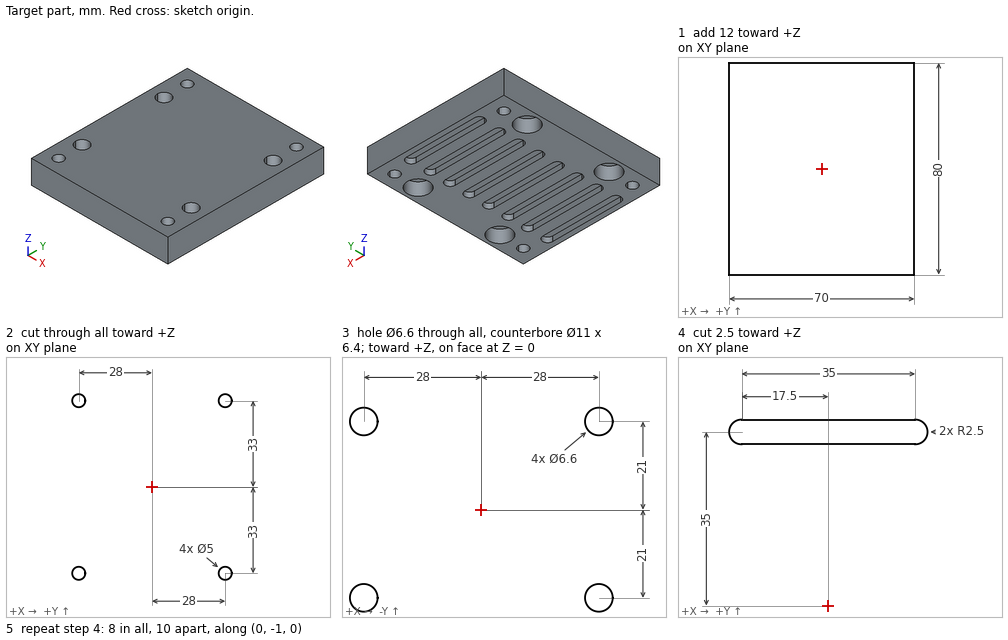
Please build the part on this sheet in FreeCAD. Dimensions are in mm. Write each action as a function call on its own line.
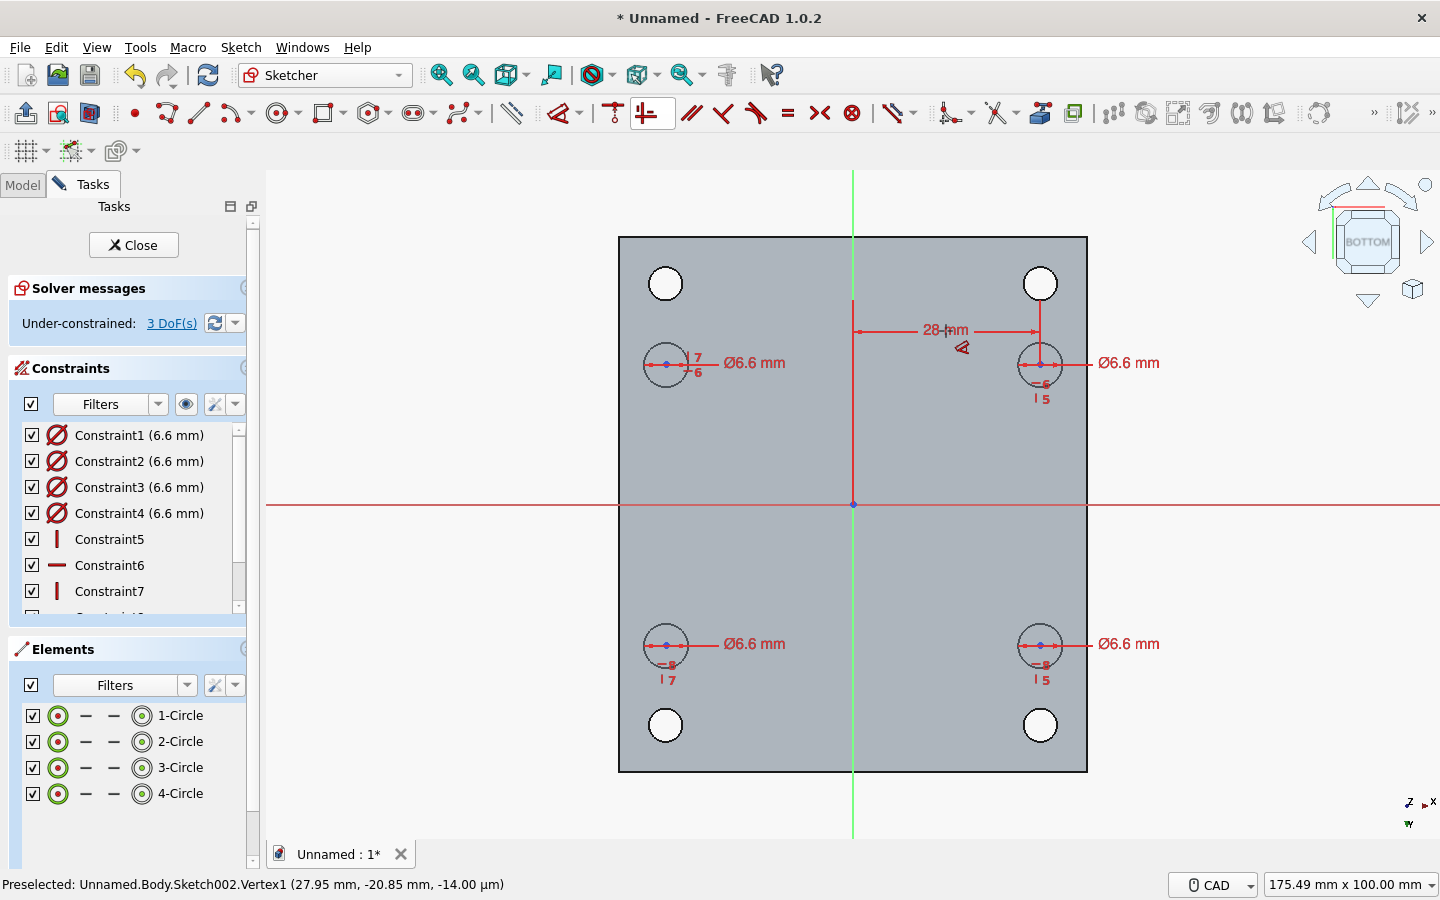
click(1040, 365)
click(1074, 435)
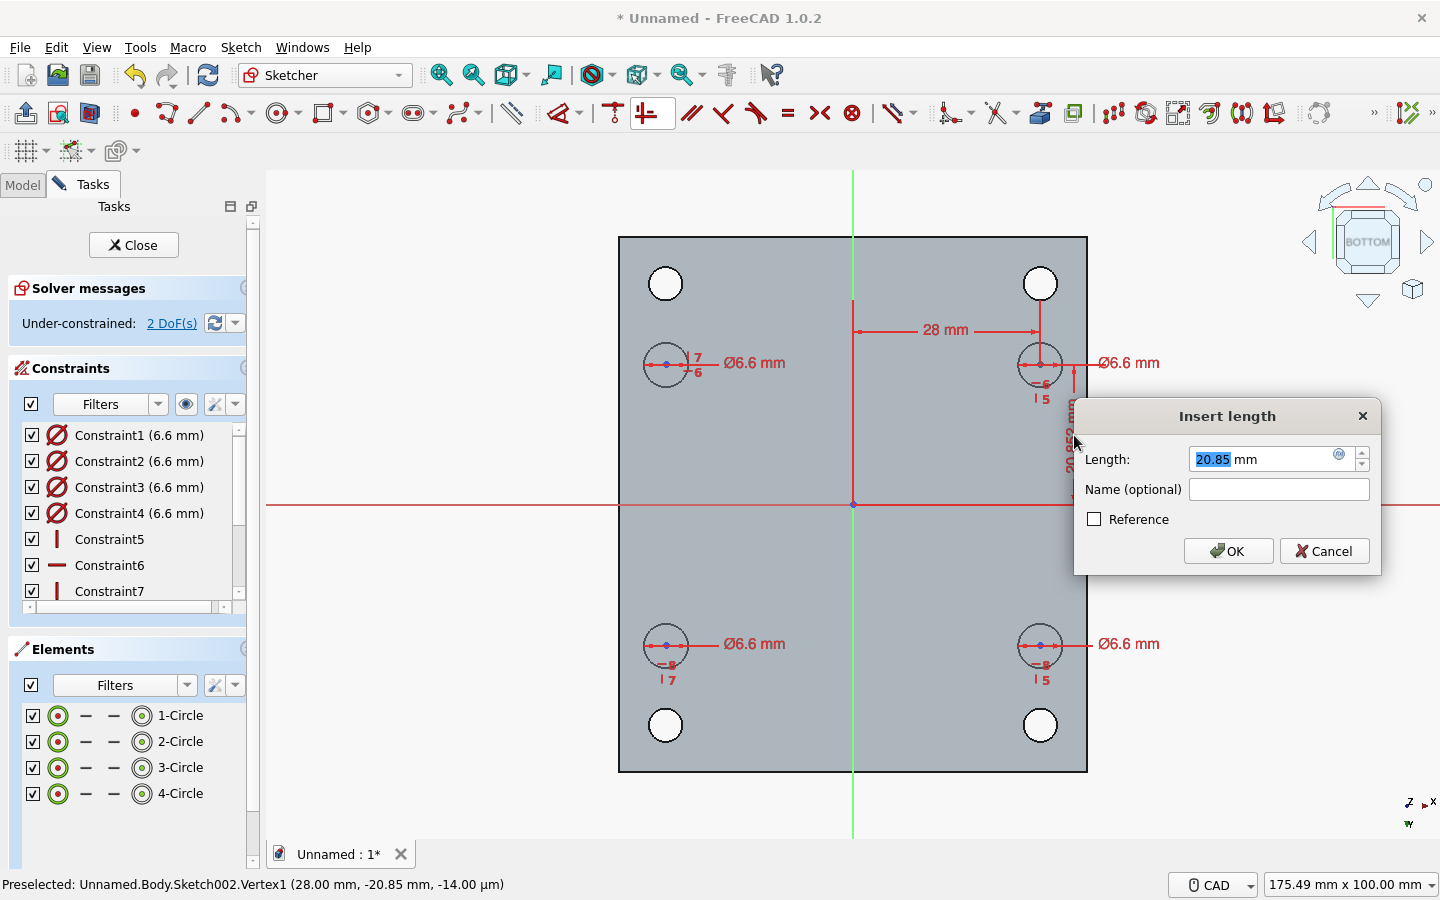
text(21)
key(Return)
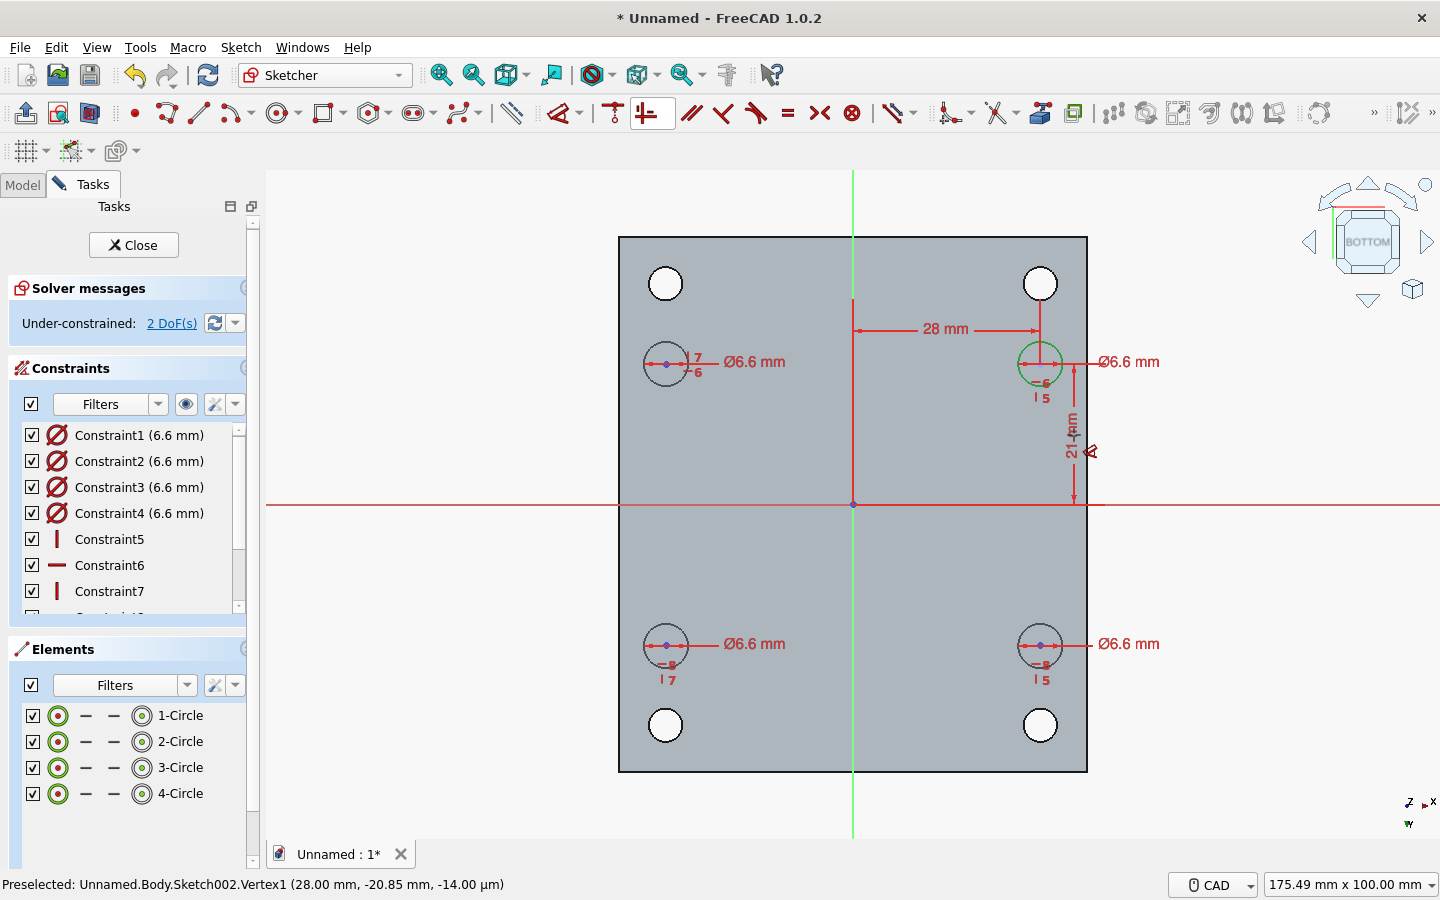
click(1040, 646)
click(1074, 575)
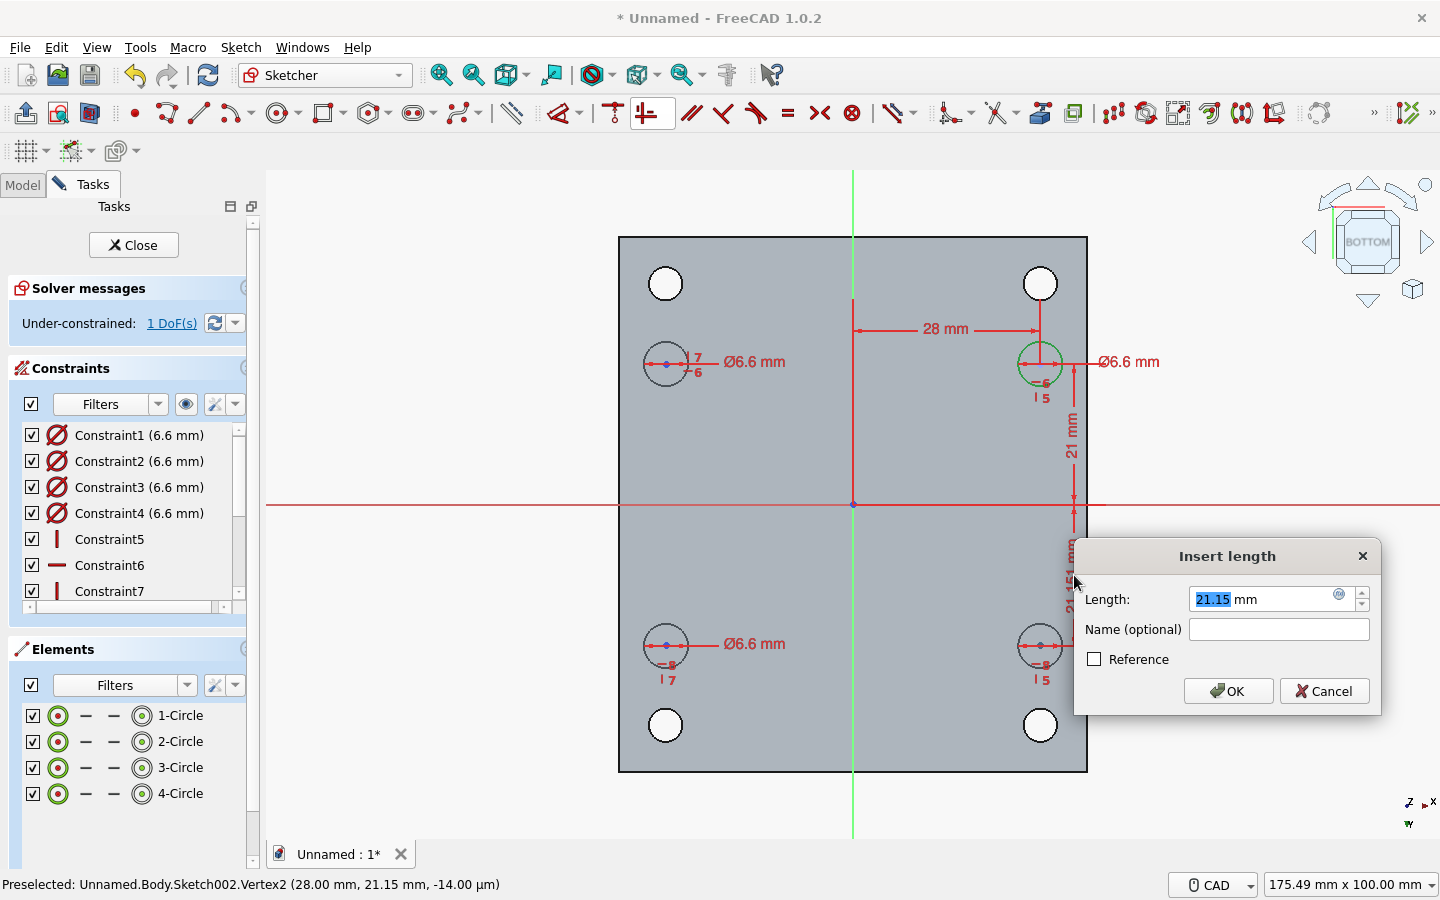
text(21)
key(Return)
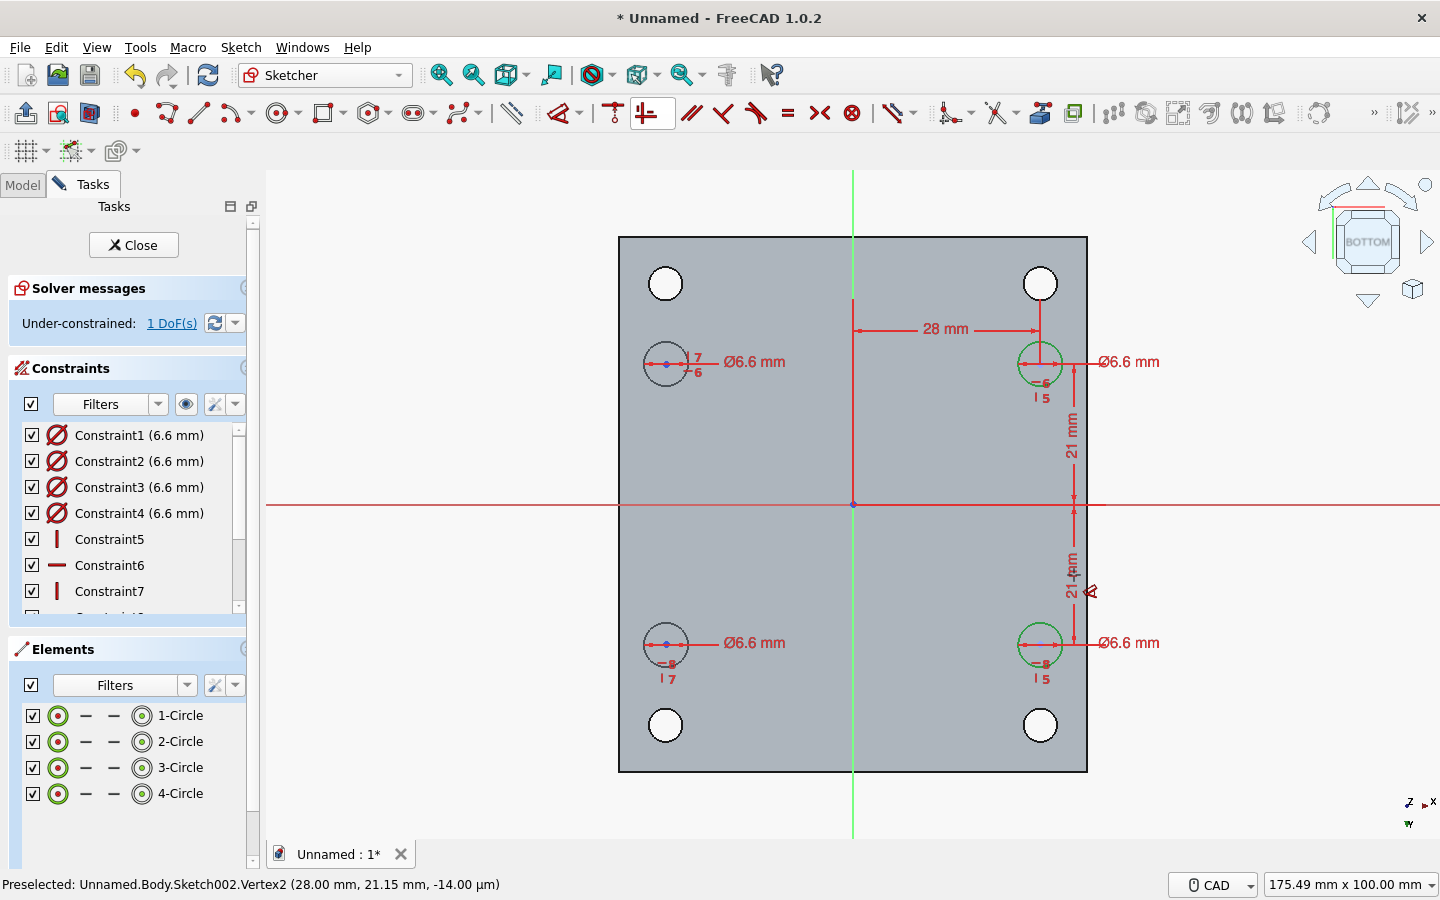
click(666, 364)
click(759, 330)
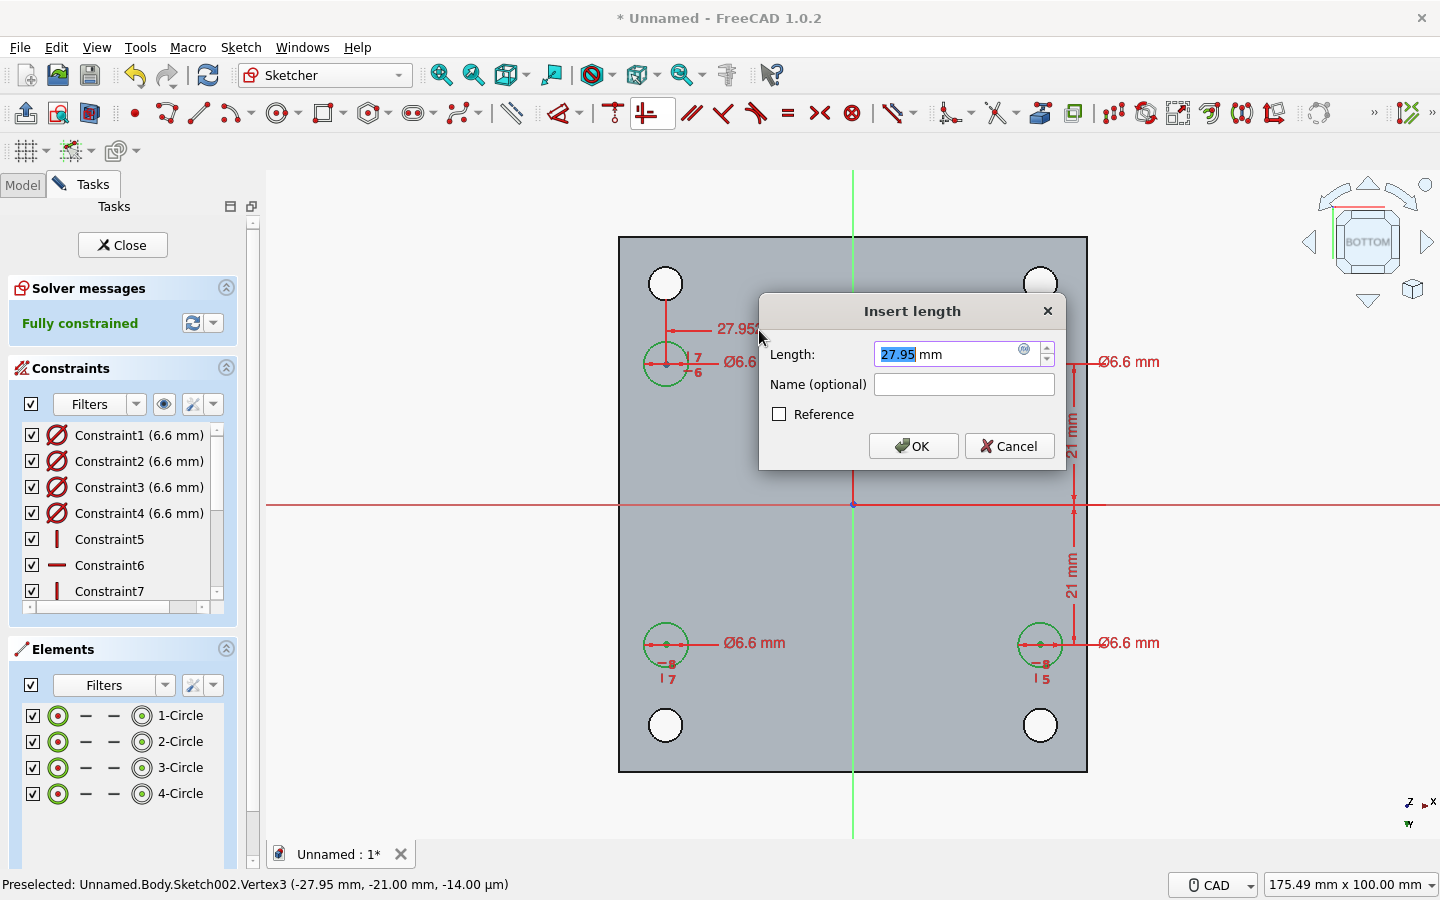
text(28)
key(Return)
key(Escape)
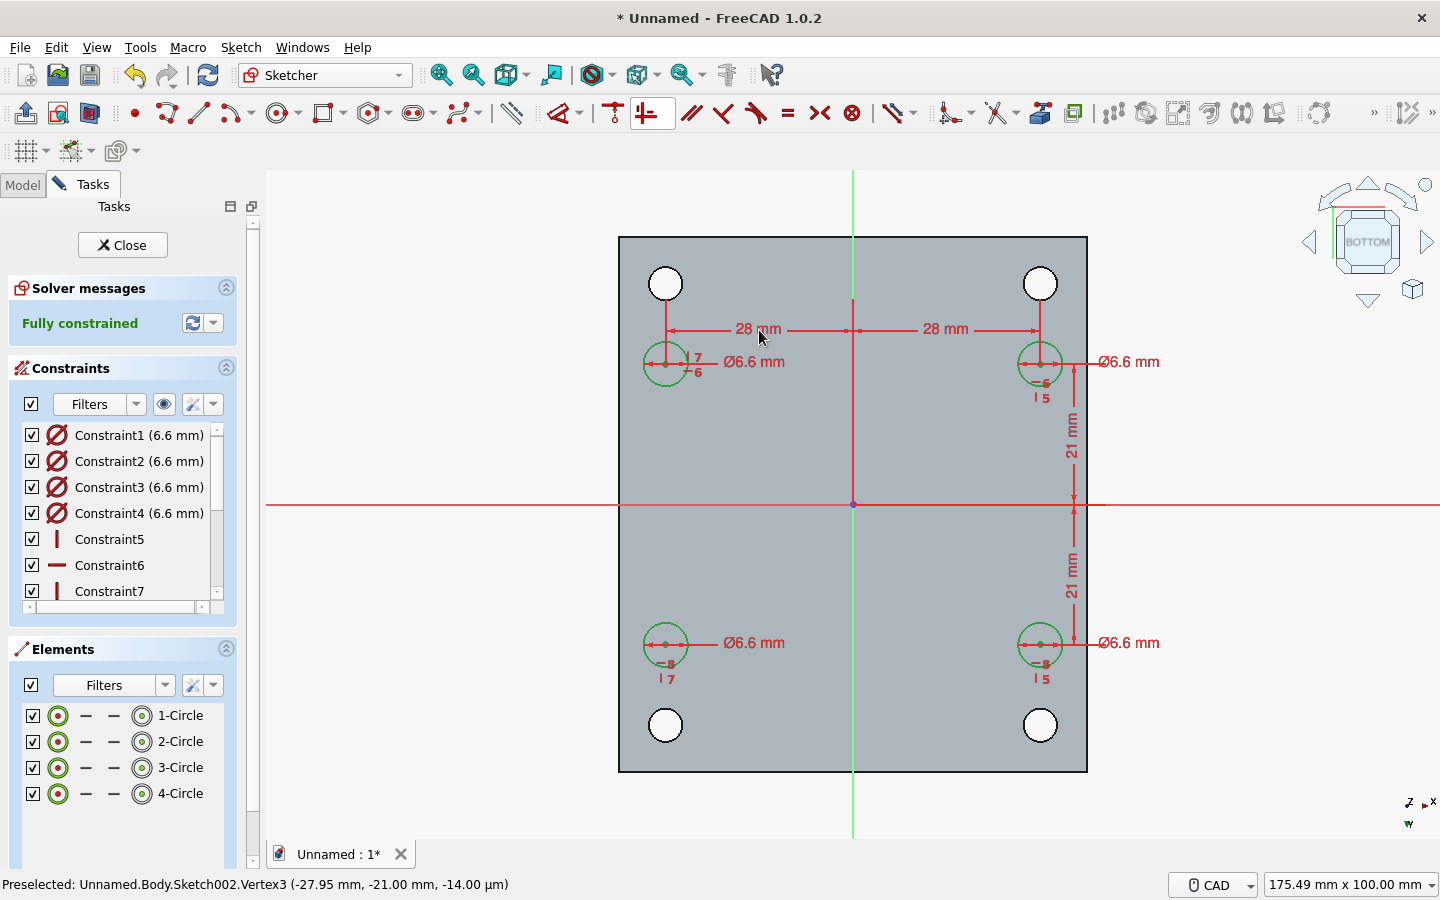
click(123, 245)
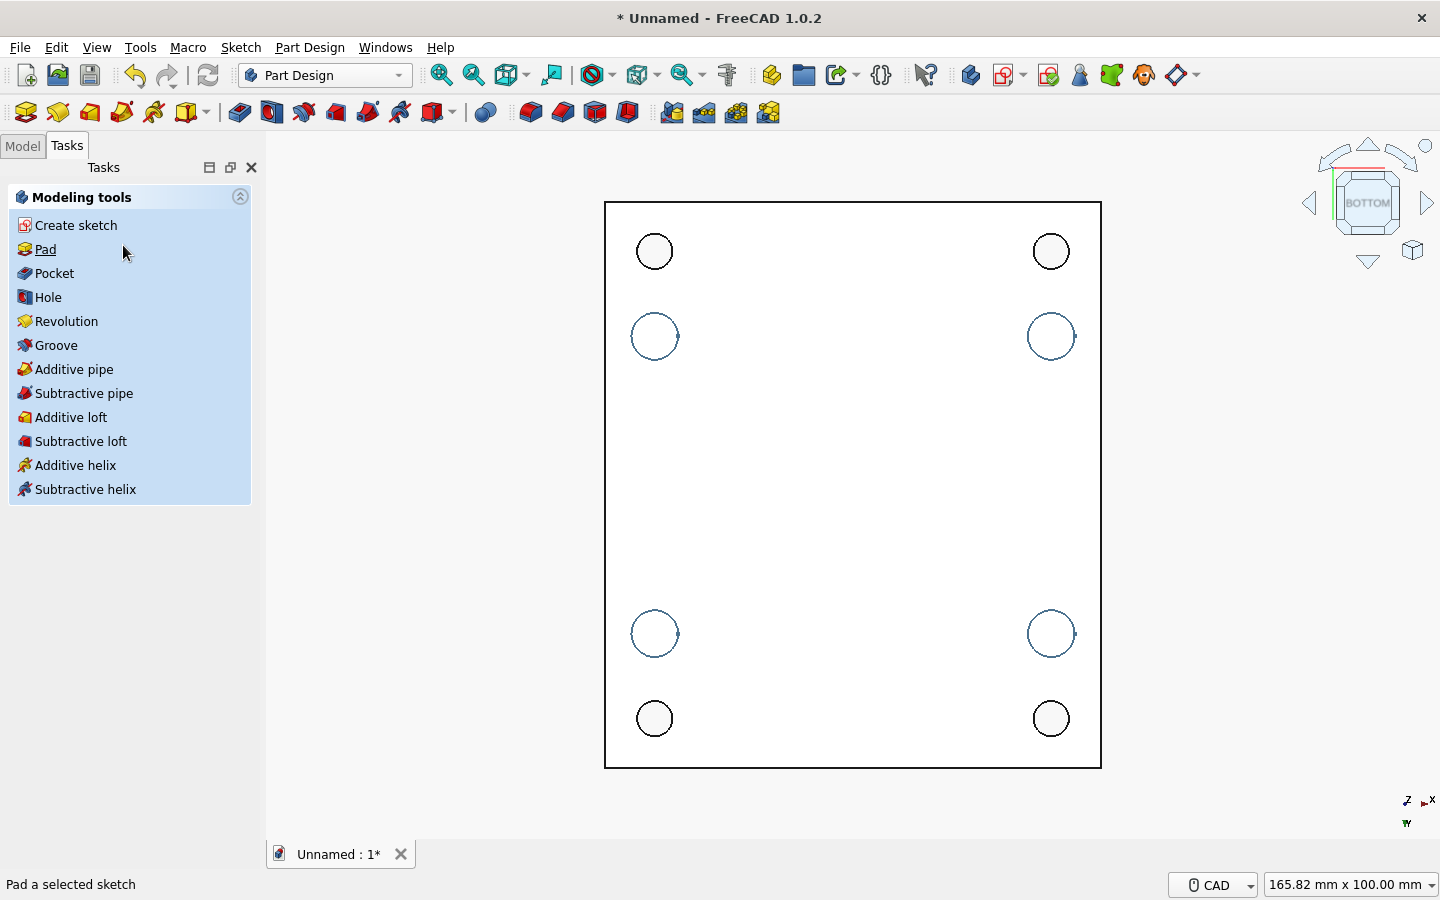
click(272, 112)